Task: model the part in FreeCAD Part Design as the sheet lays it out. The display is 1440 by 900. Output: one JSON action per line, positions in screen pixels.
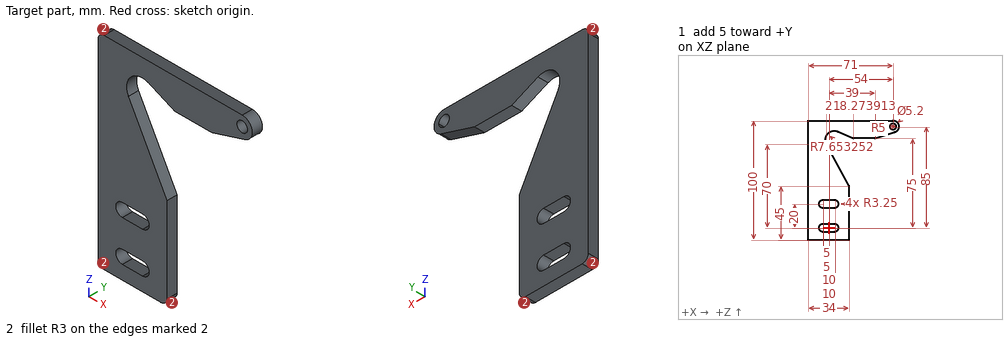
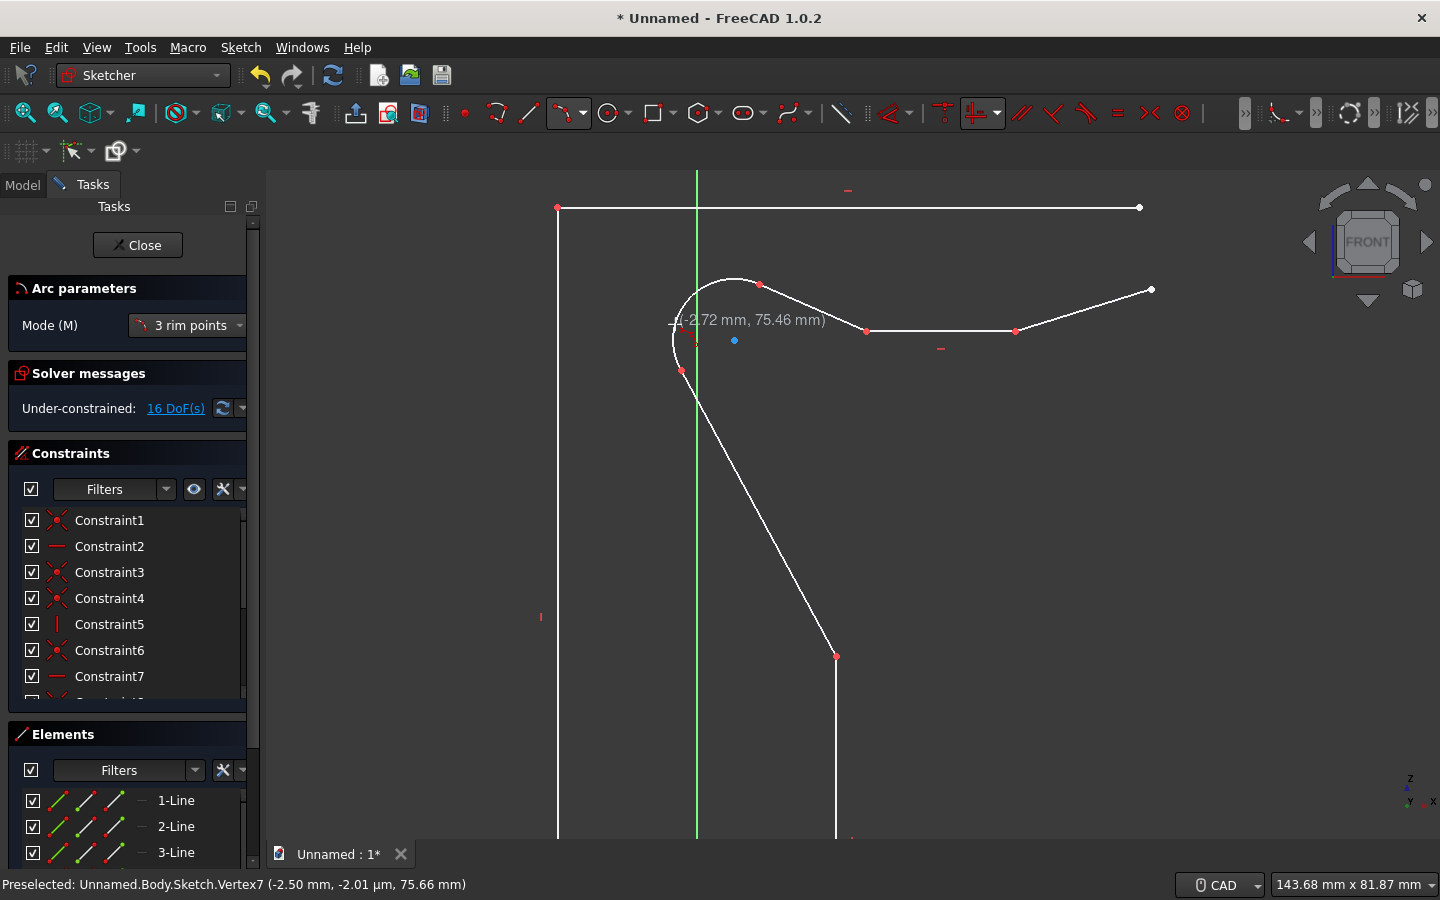
{"action": "left_click", "coordinate": [1139, 208]}
{"action": "left_click", "coordinate": [1152, 289]}
{"action": "left_click", "coordinate": [1179, 241]}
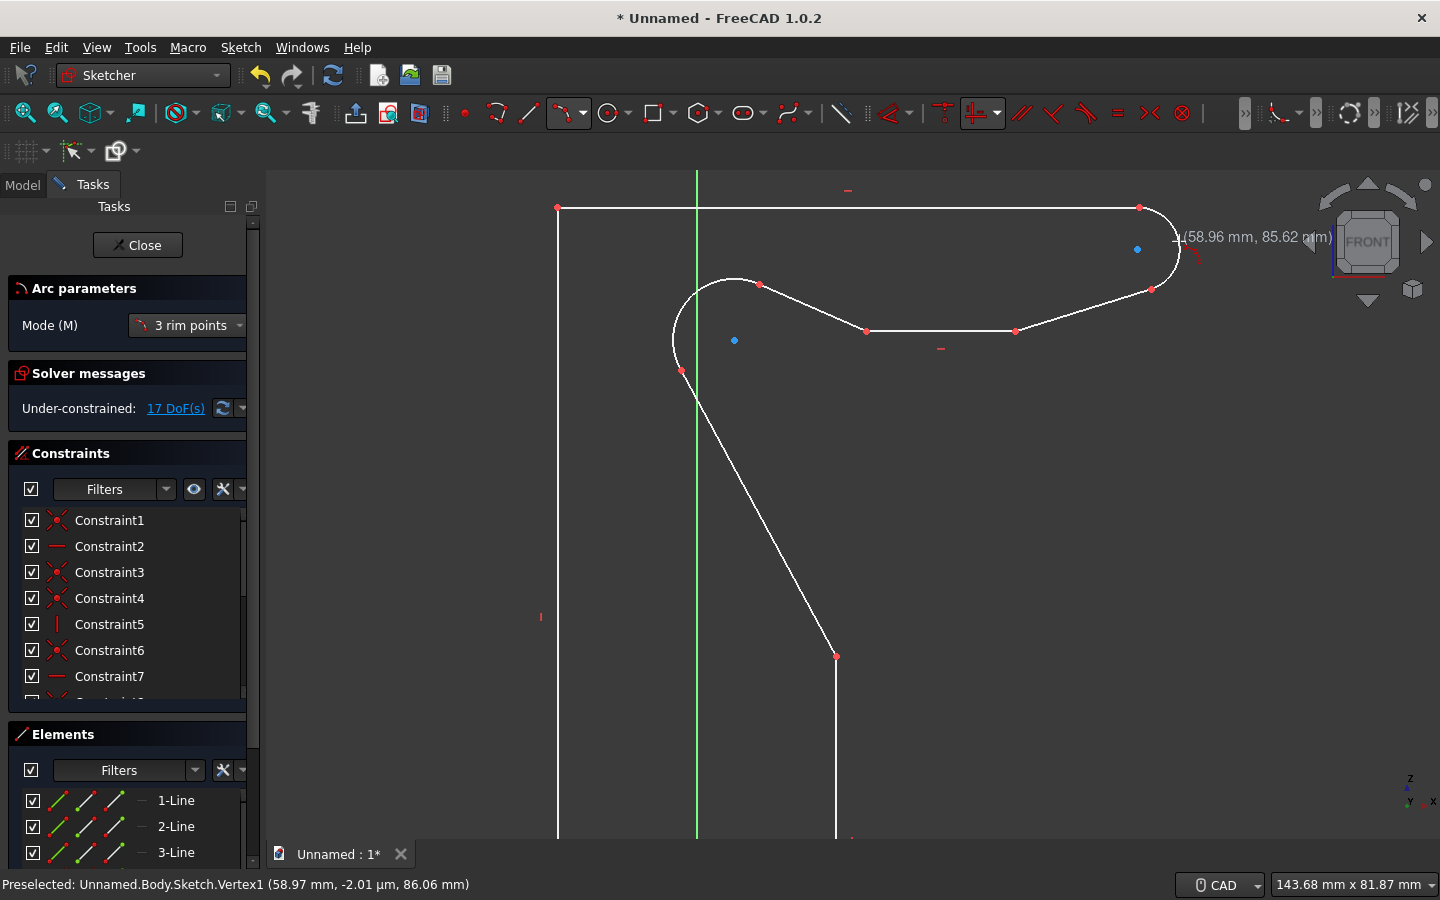
{"action": "key", "text": "g s"}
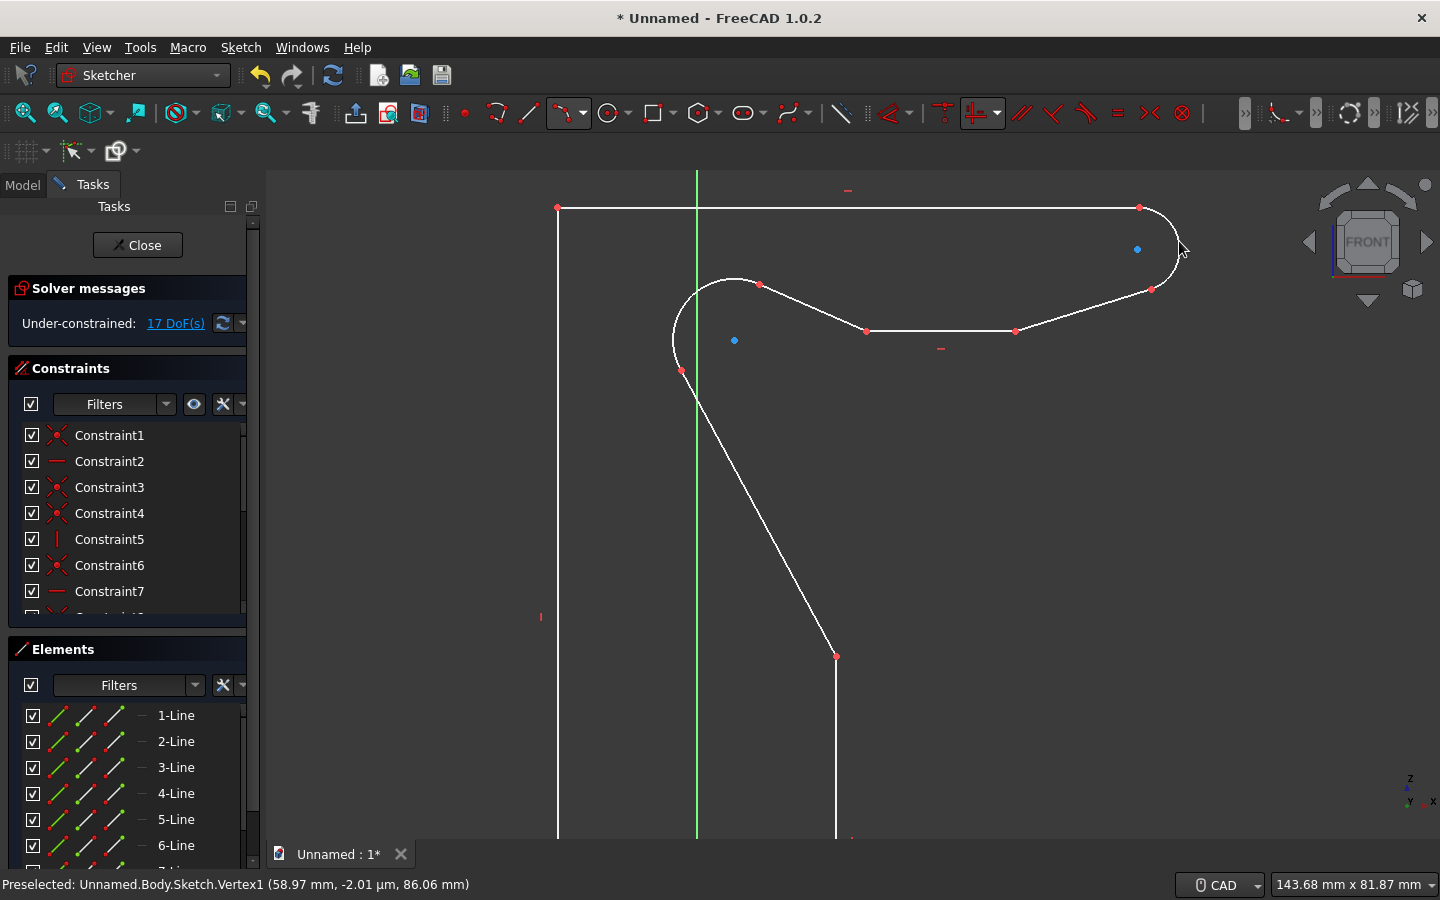
{"action": "left_click", "coordinate": [656, 778]}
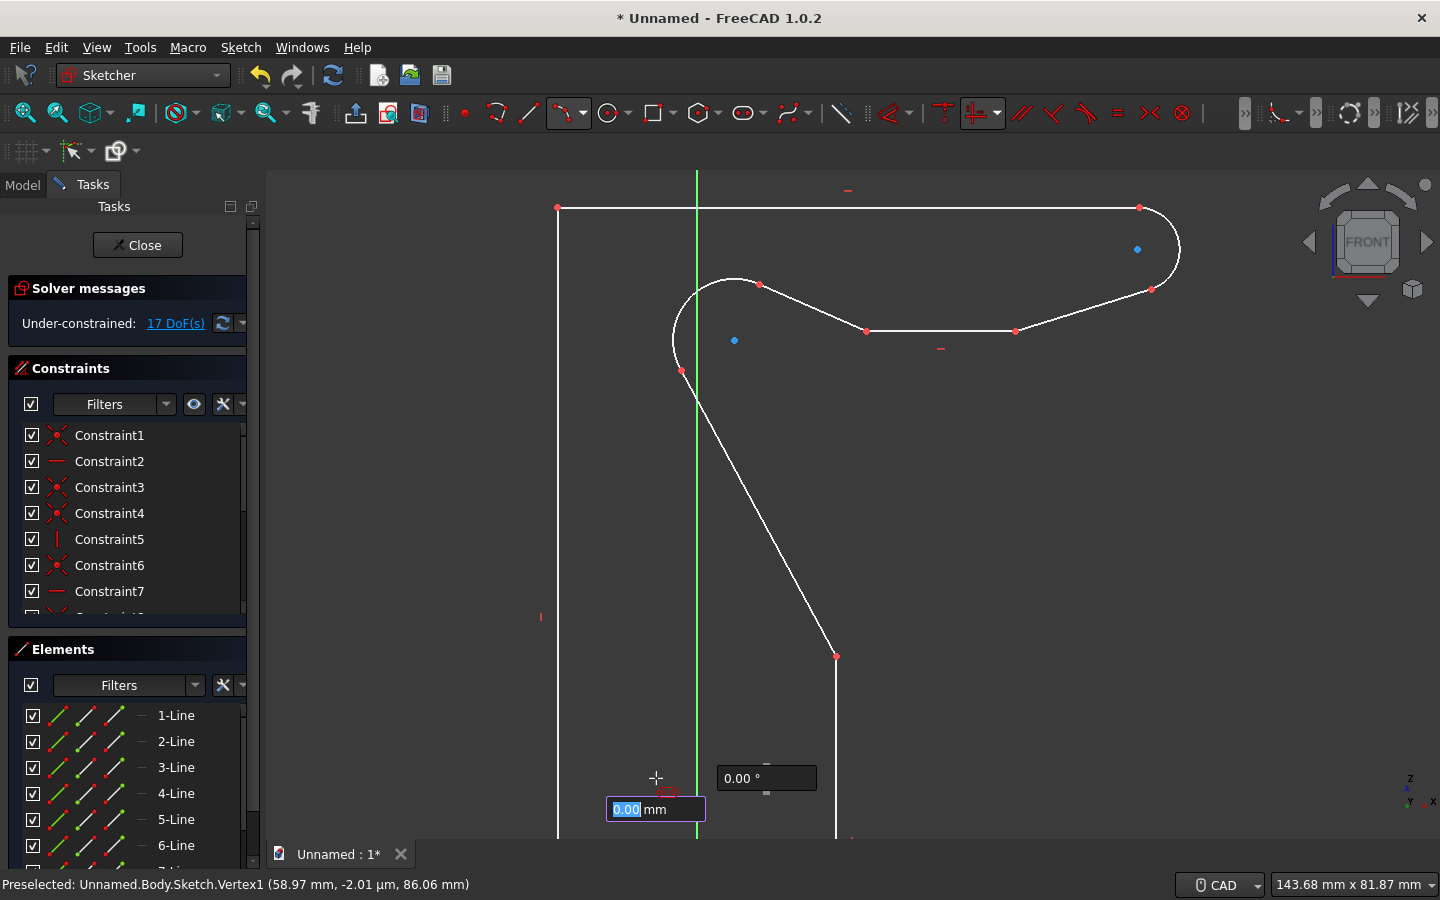
{"action": "left_click", "coordinate": [738, 778]}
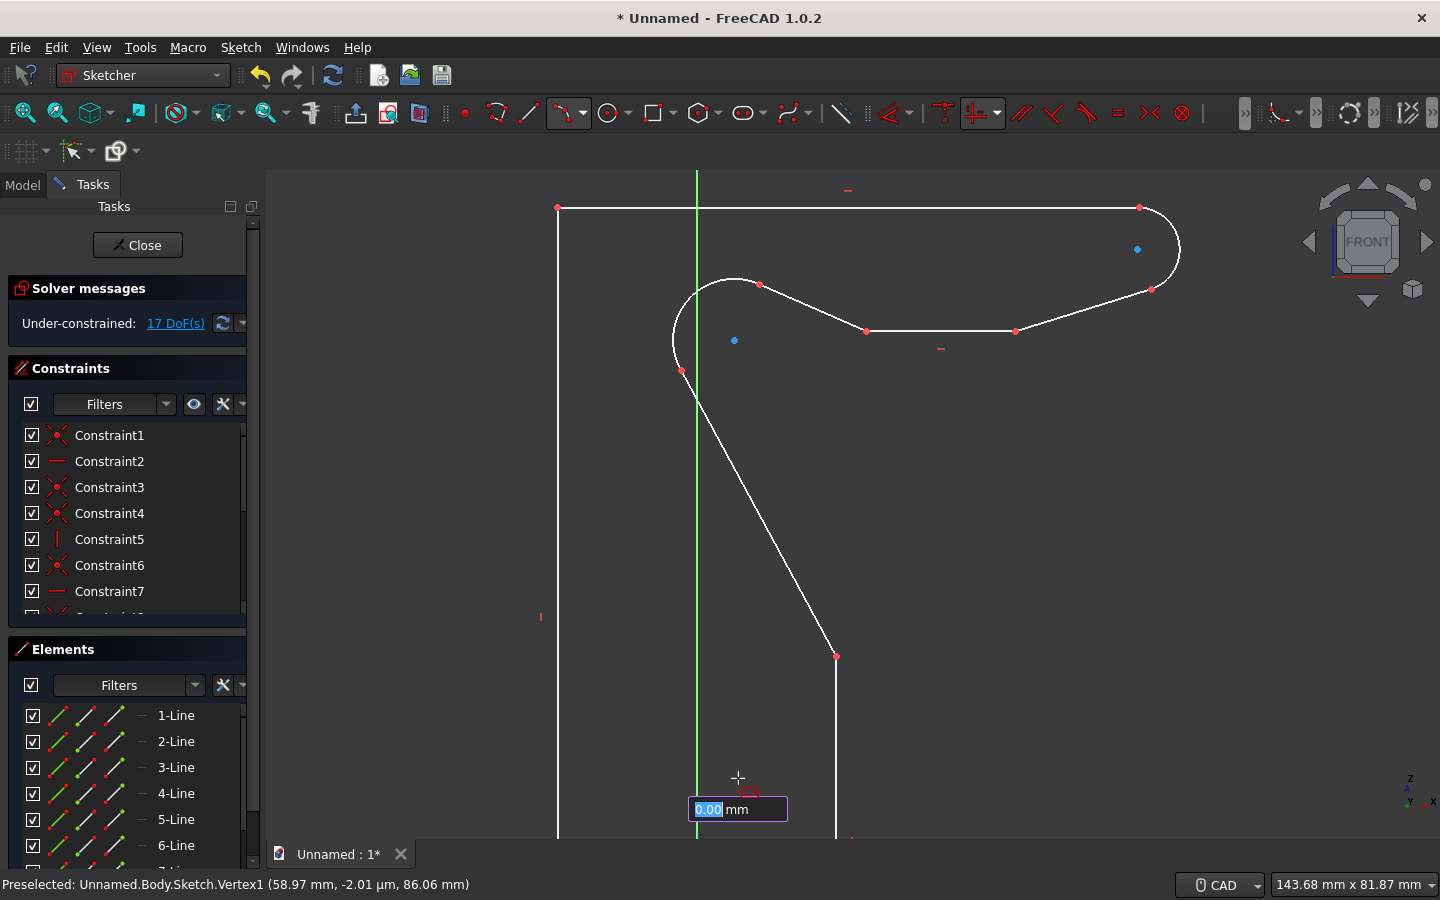
{"action": "scroll", "coordinate": [709, 752], "scroll_direction": "up", "scroll_amount": 2}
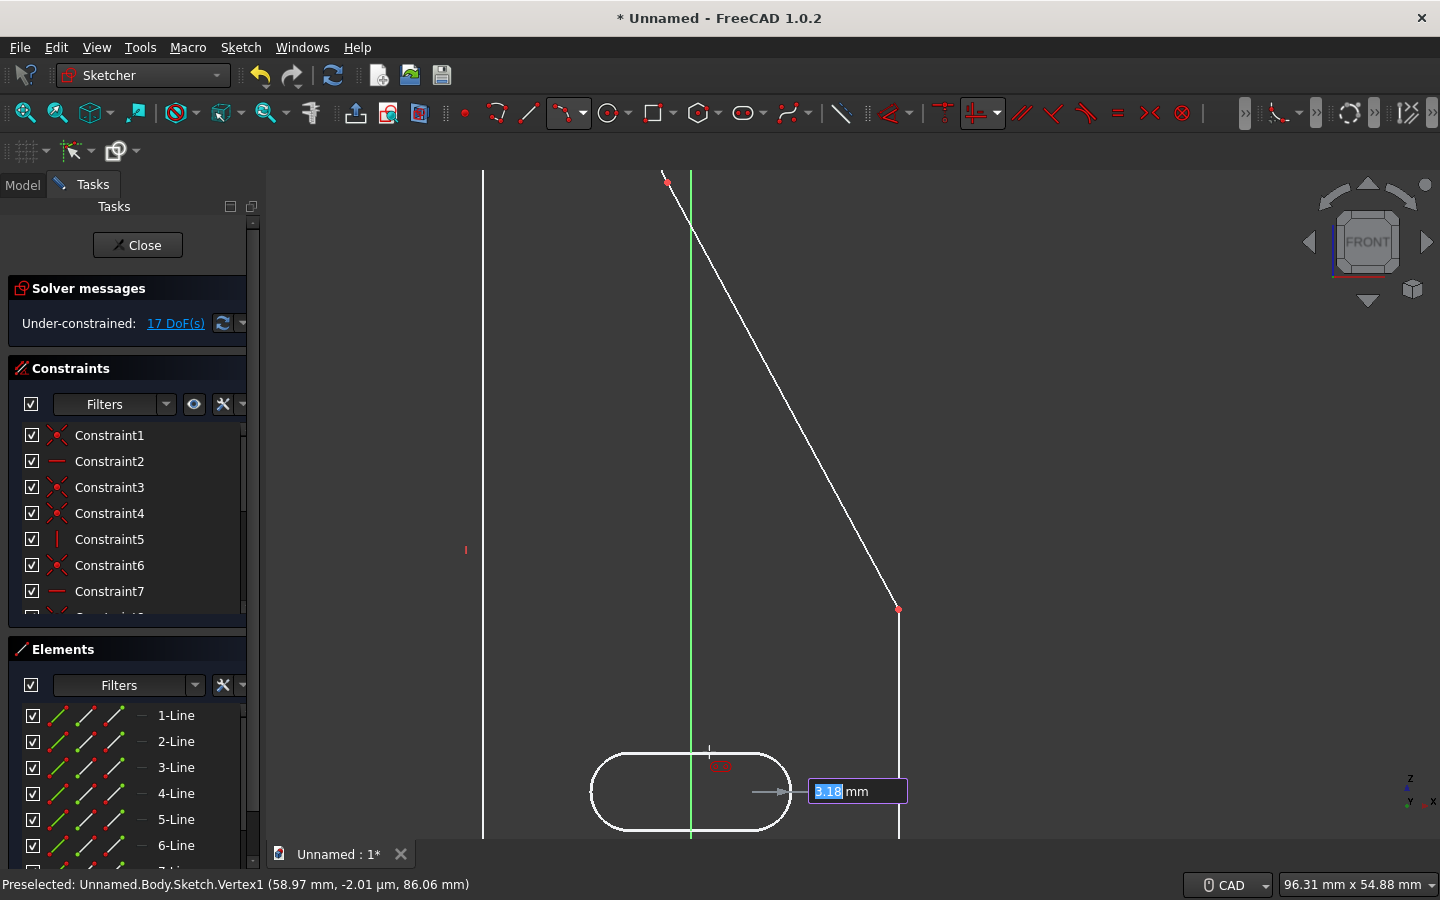
{"action": "left_click", "coordinate": [709, 751]}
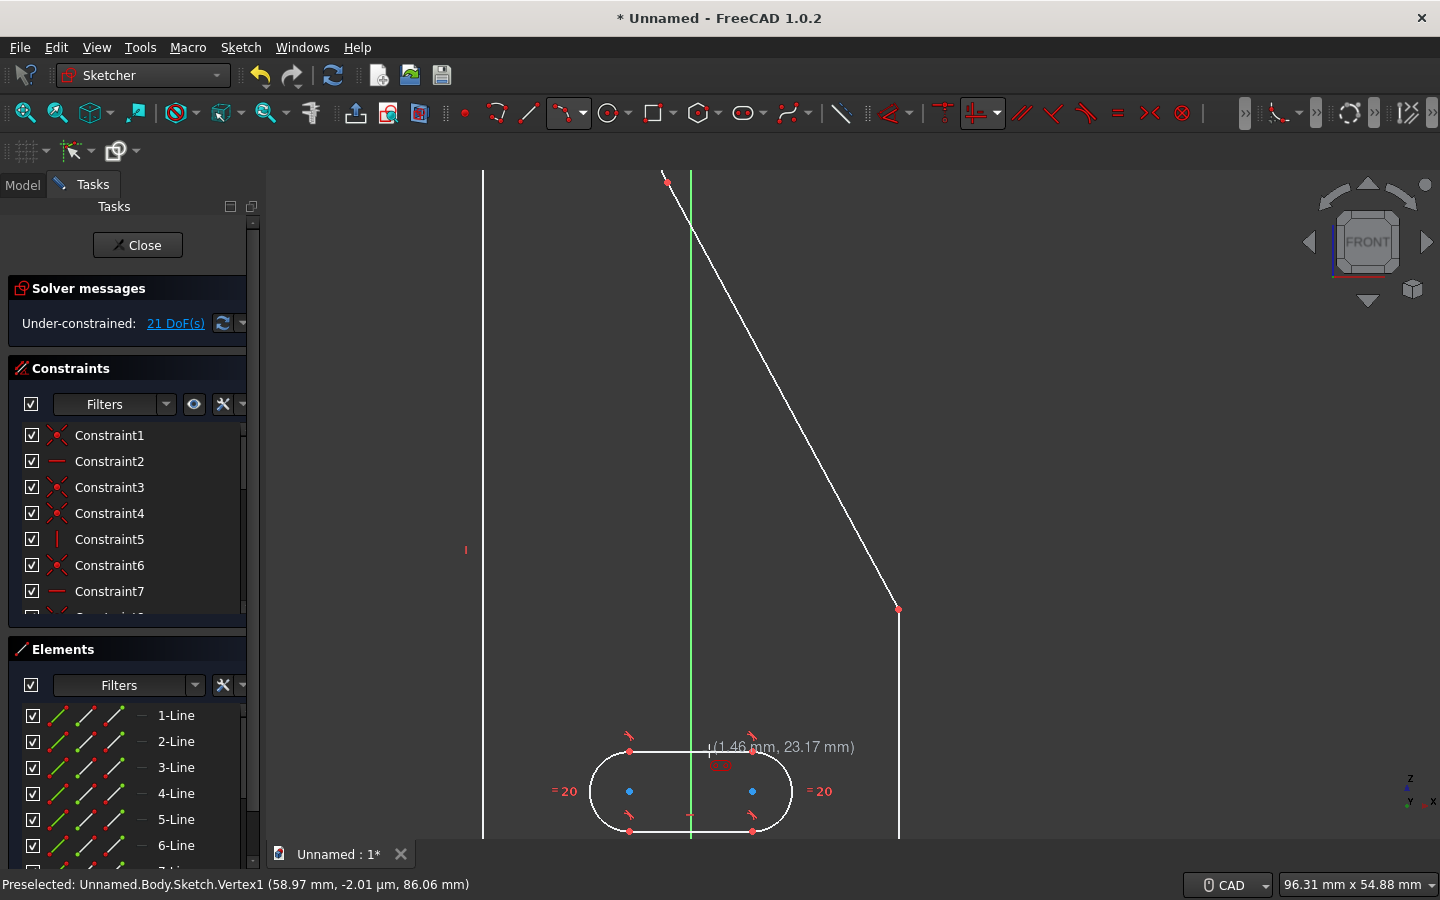
{"action": "scroll", "coordinate": [690, 480], "scroll_direction": "down", "scroll_amount": 5}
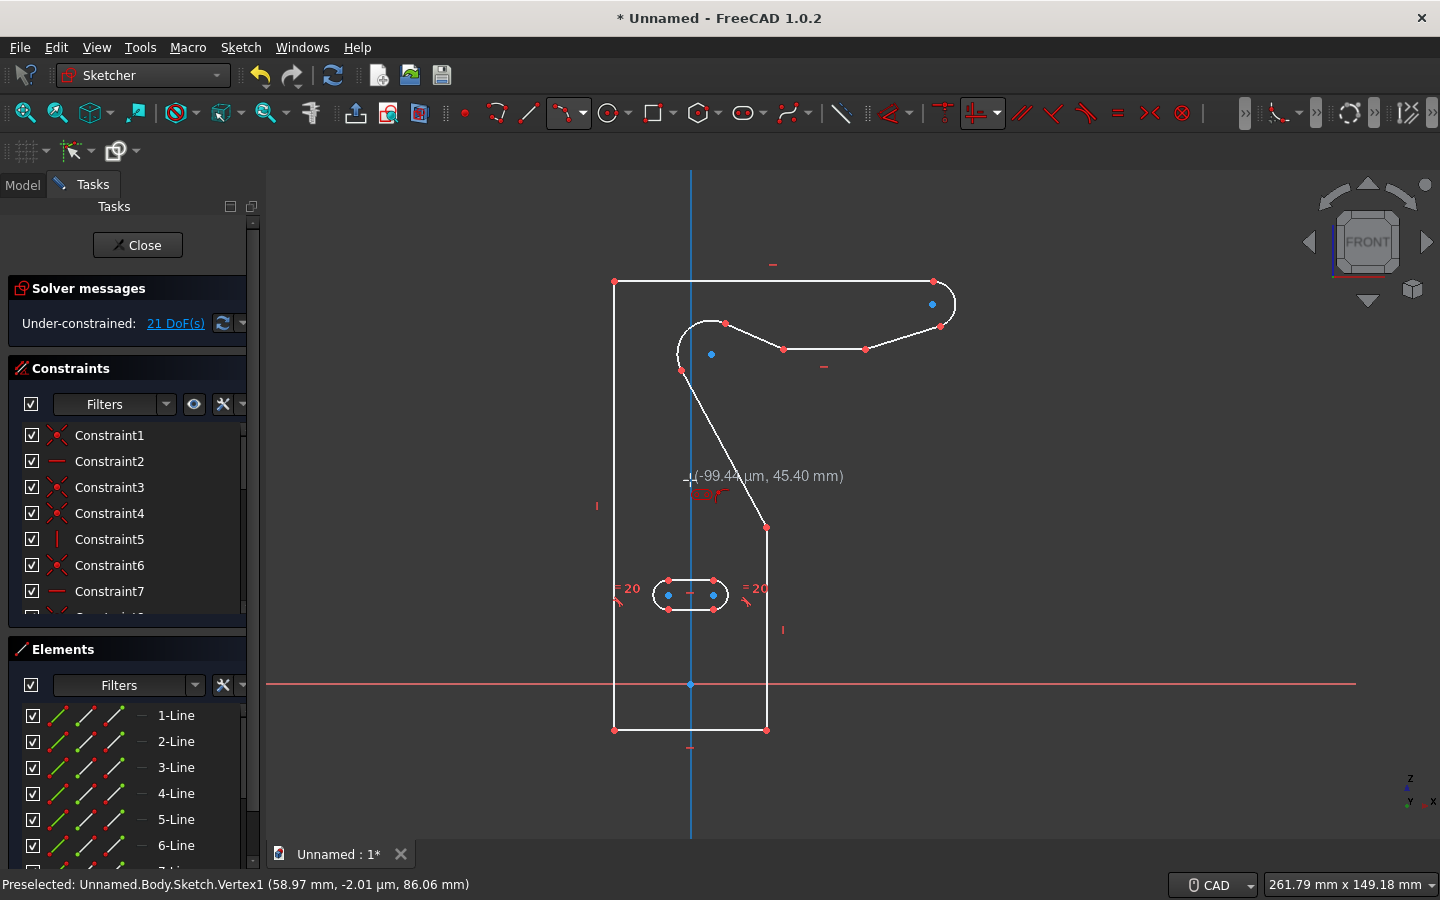
{"action": "scroll", "coordinate": [668, 684], "scroll_direction": "up", "scroll_amount": 3}